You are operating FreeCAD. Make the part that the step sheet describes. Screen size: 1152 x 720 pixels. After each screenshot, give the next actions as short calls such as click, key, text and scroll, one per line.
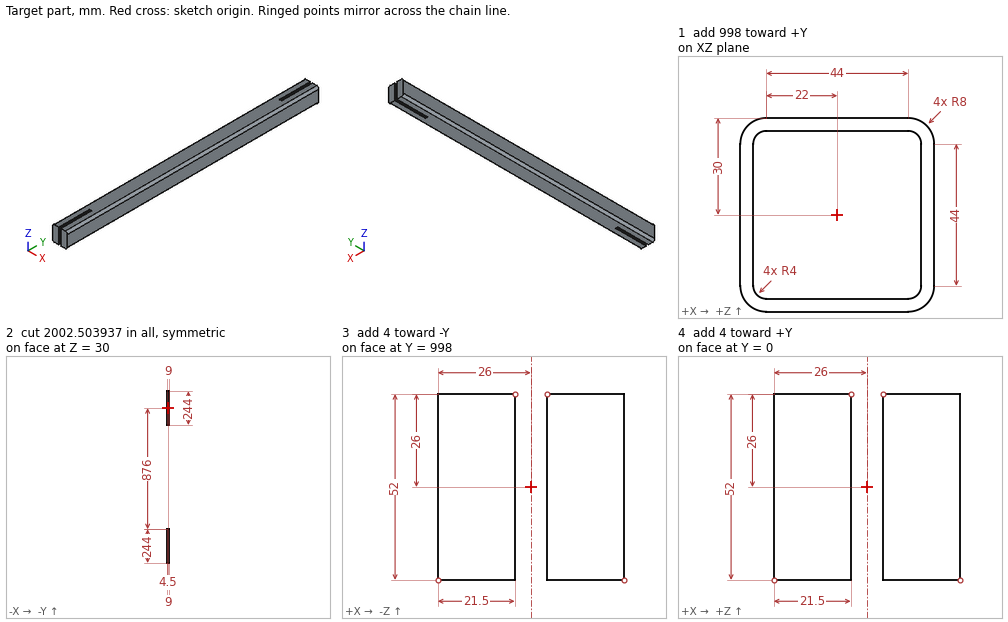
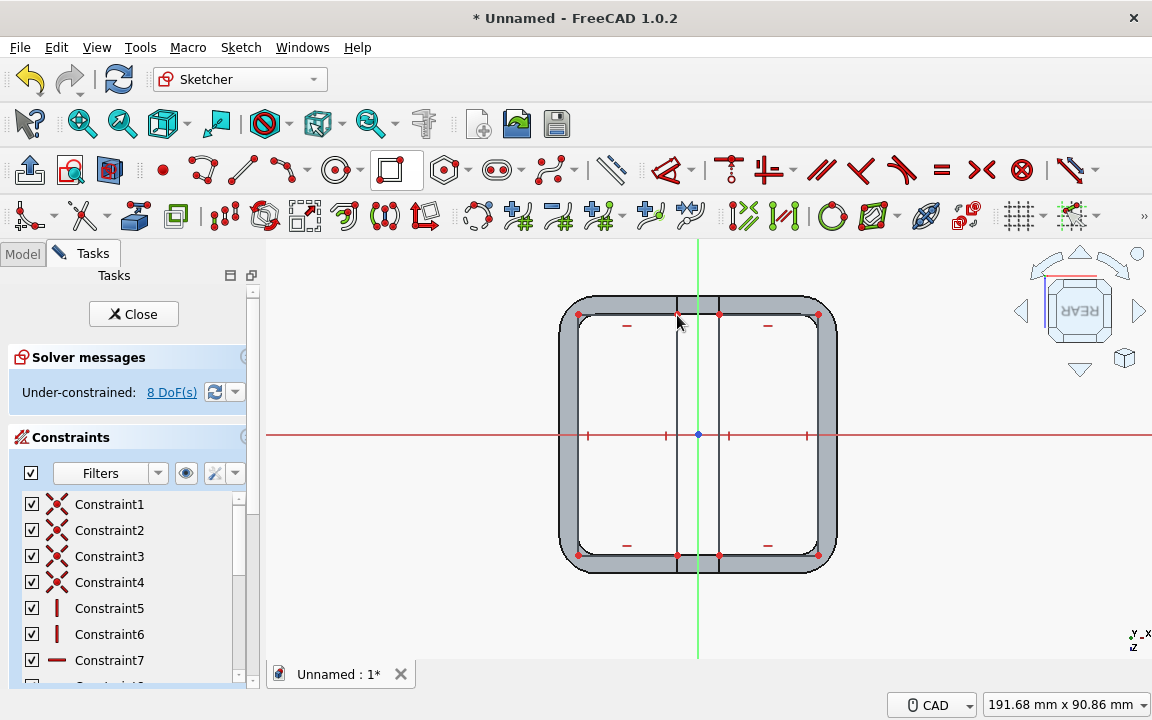
click(719, 315)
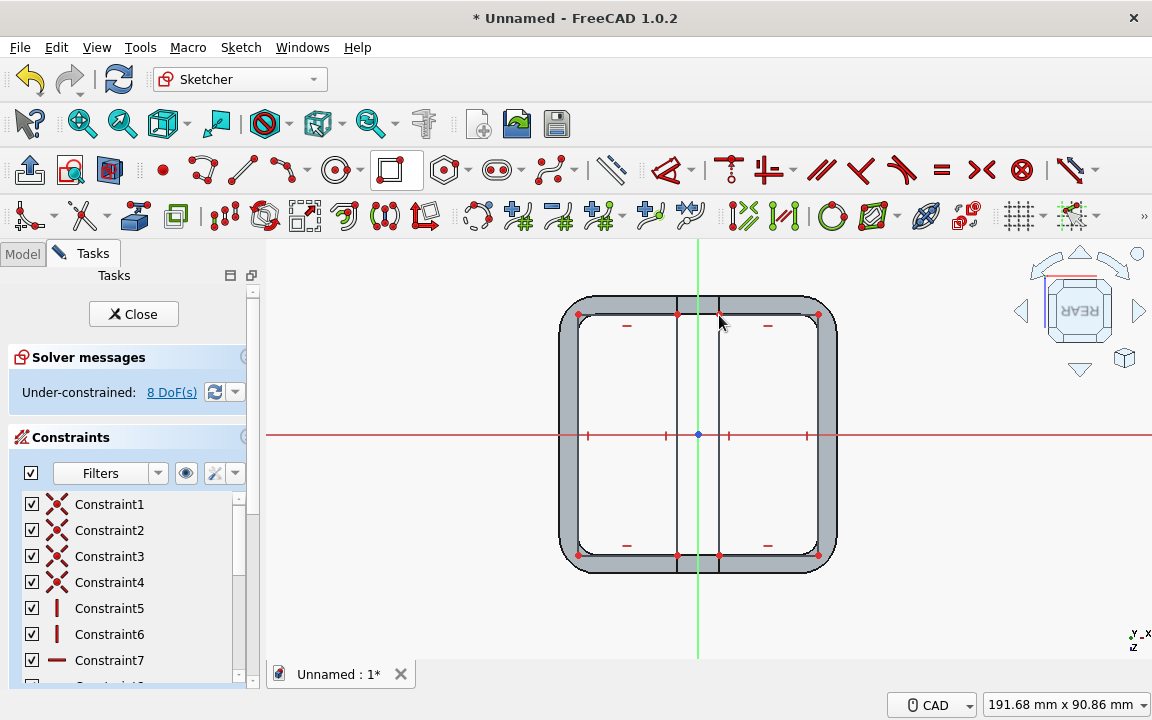
click(698, 605)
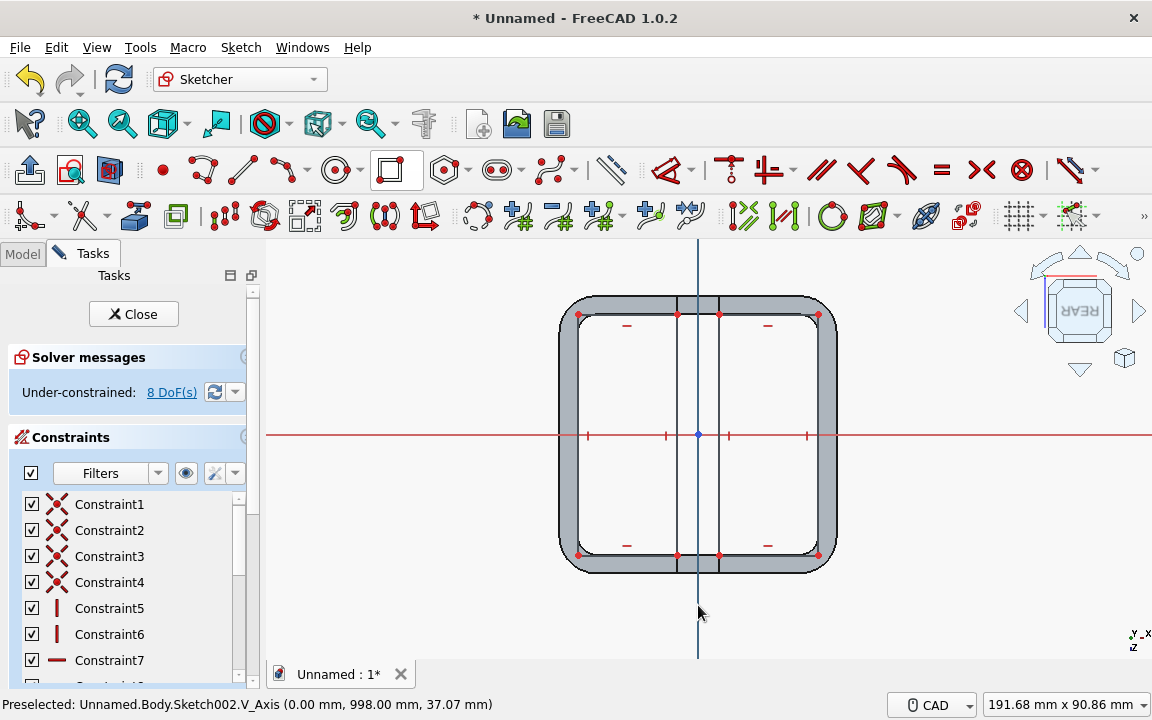
click(982, 170)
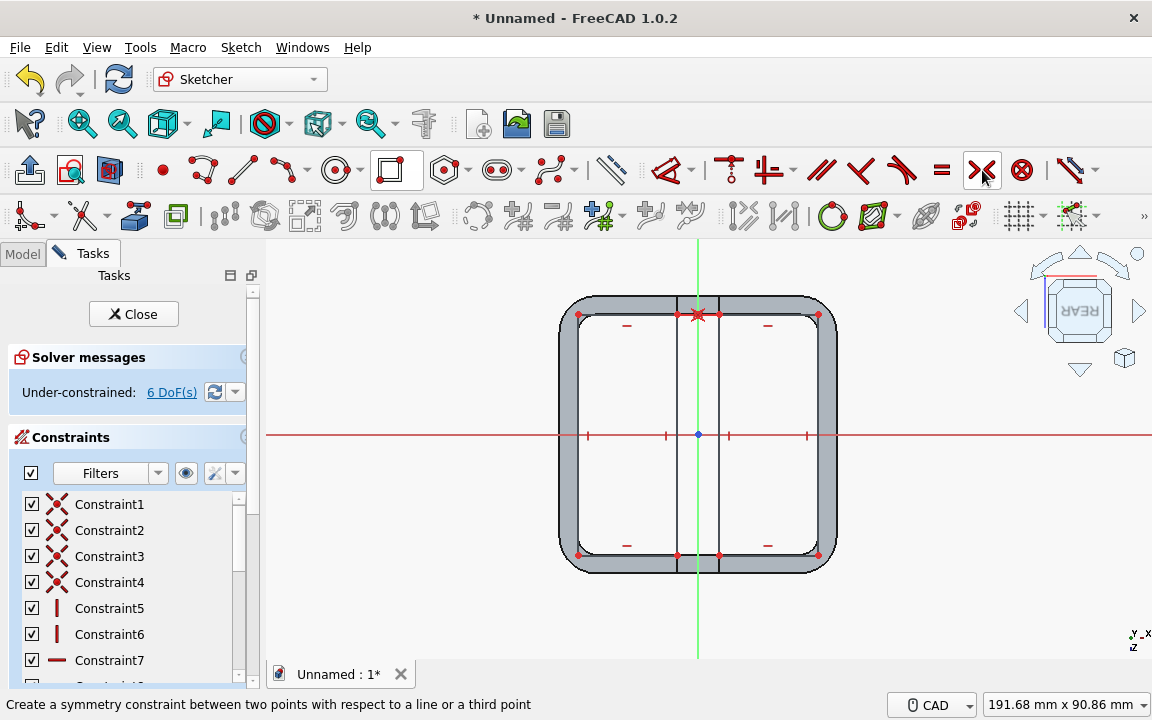
click(578, 556)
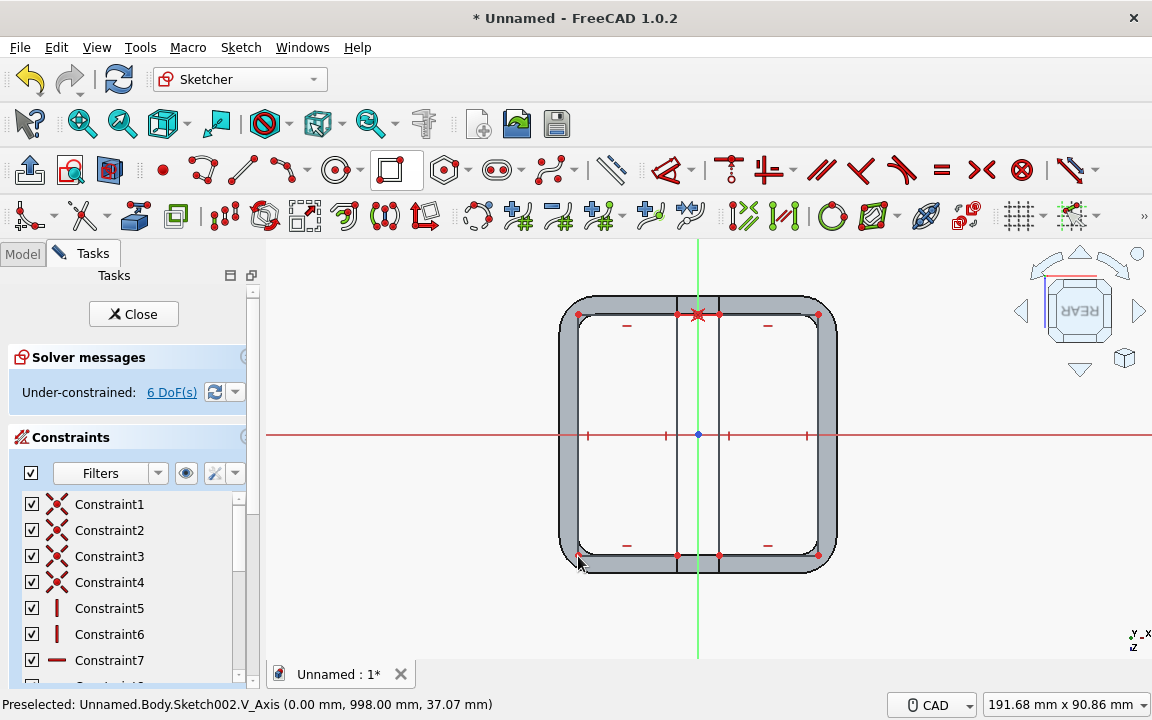
click(818, 556)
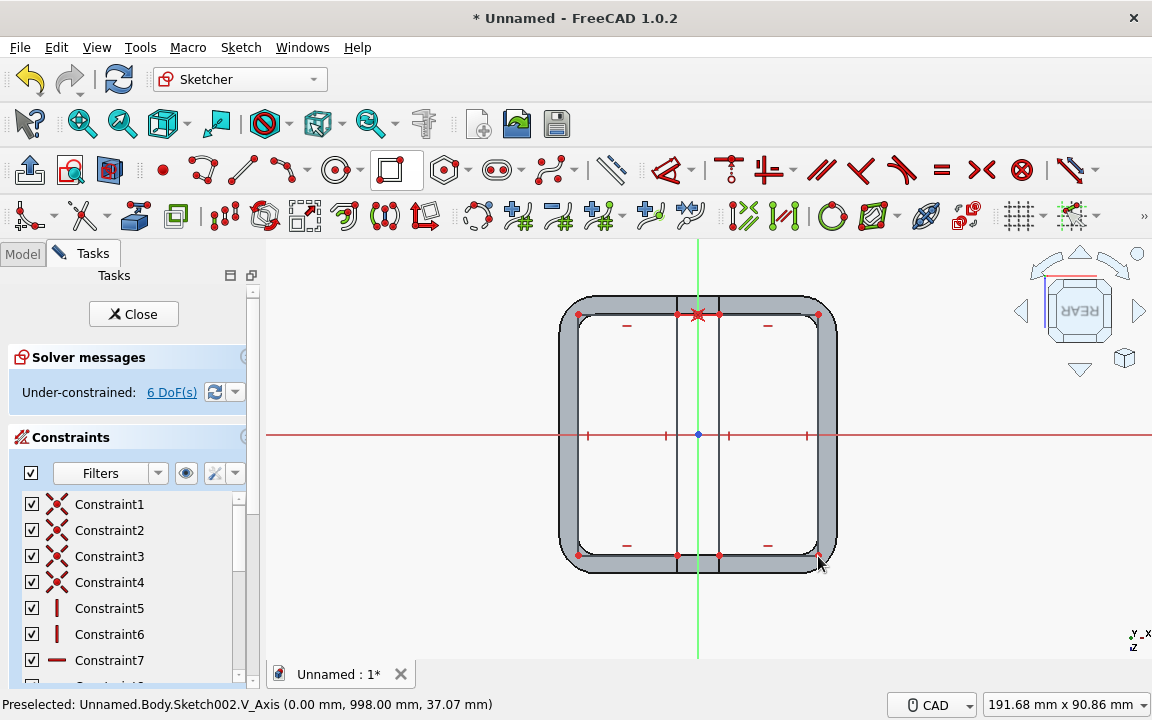
click(698, 605)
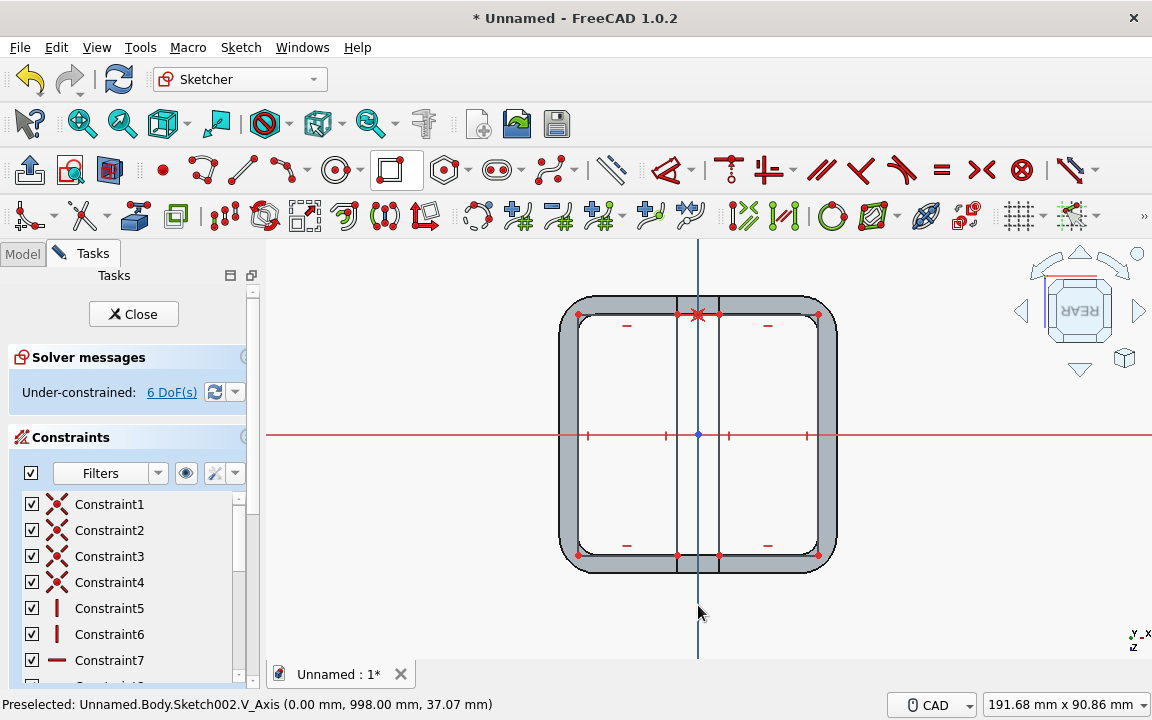
click(982, 170)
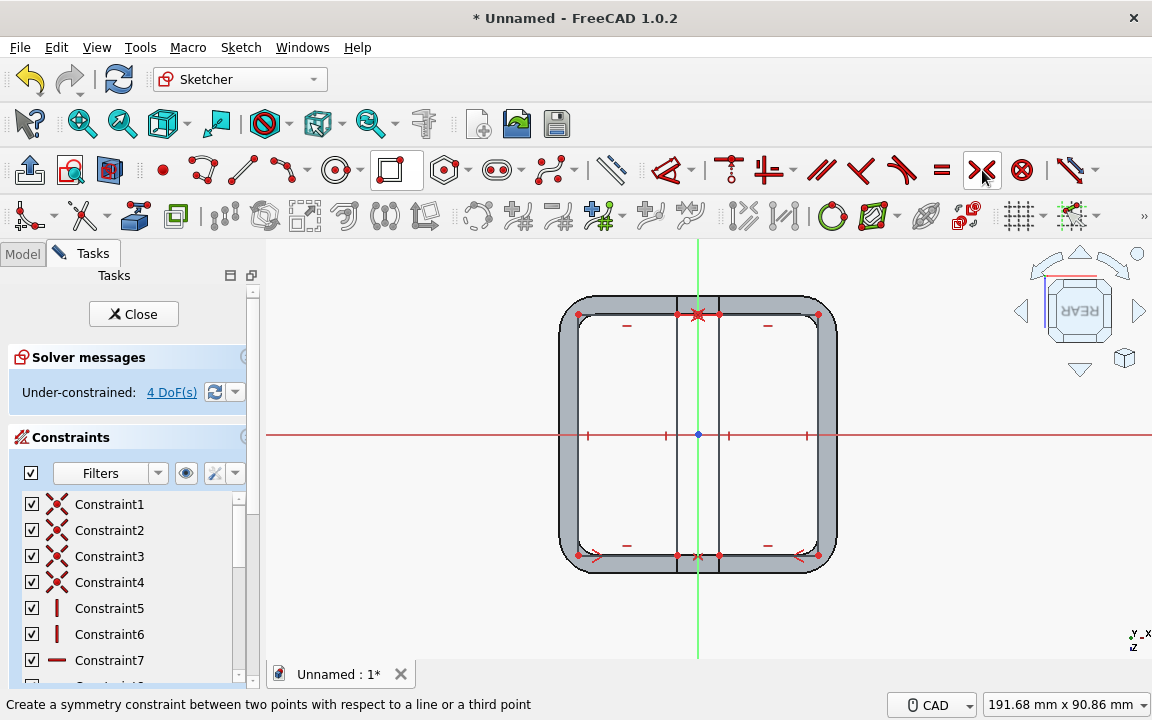
click(666, 170)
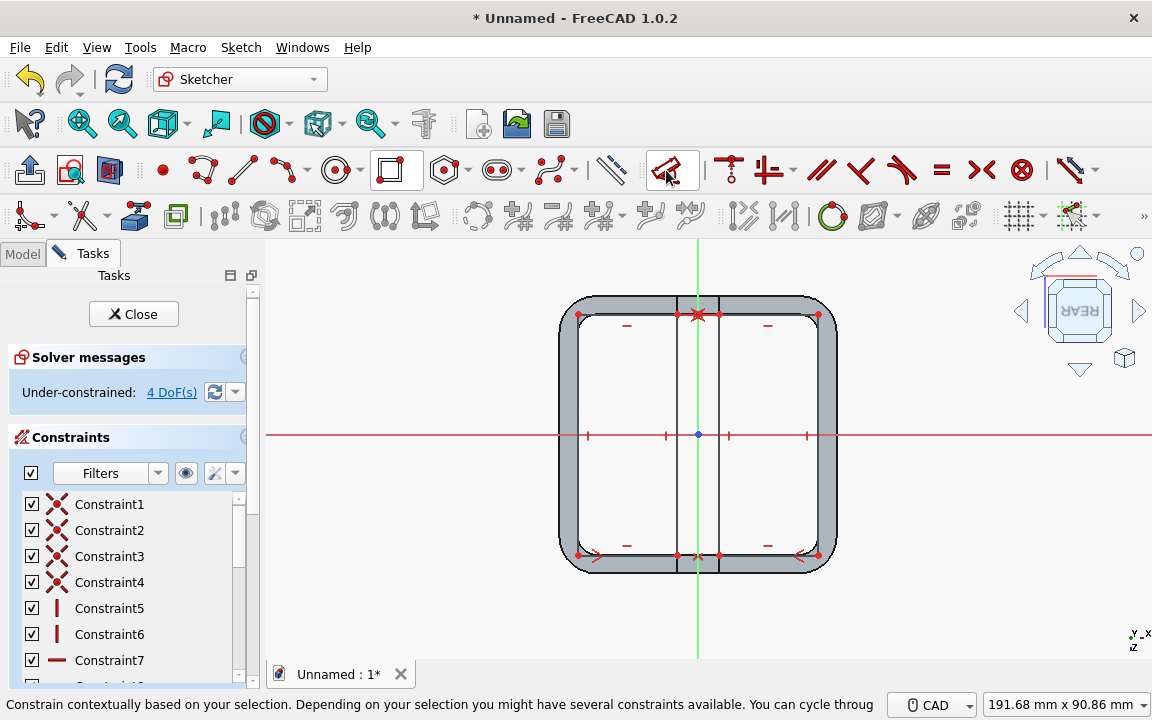
click(578, 387)
click(544, 380)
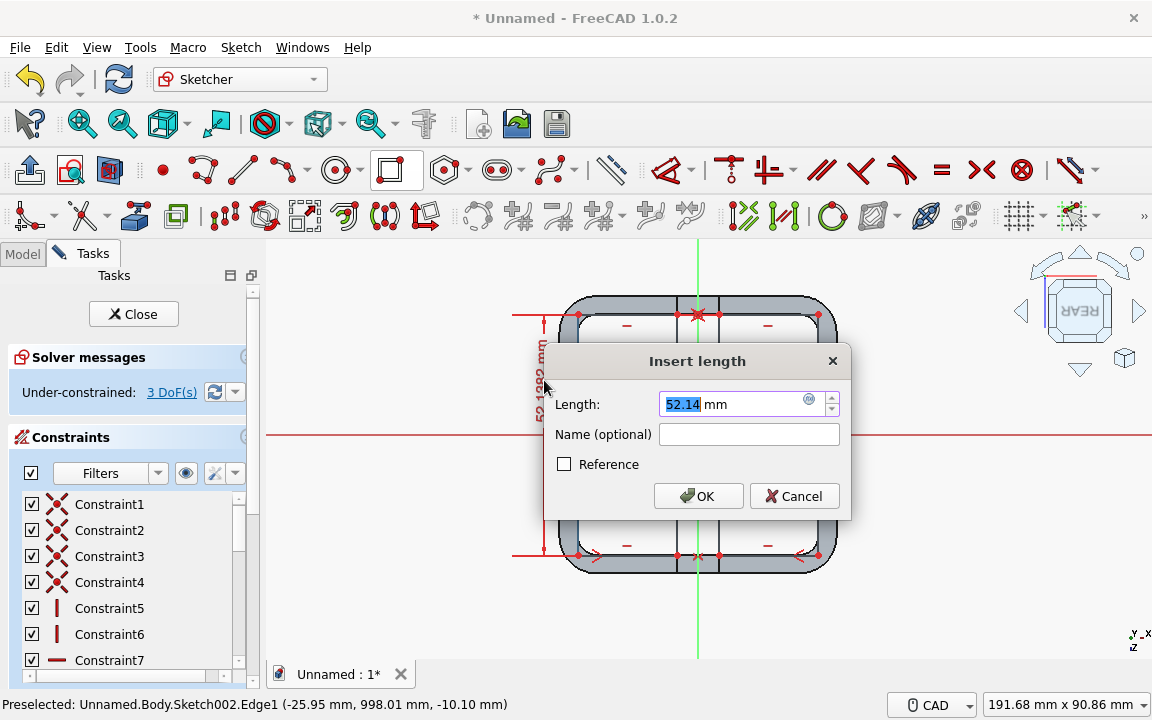
text(52)
key(Return)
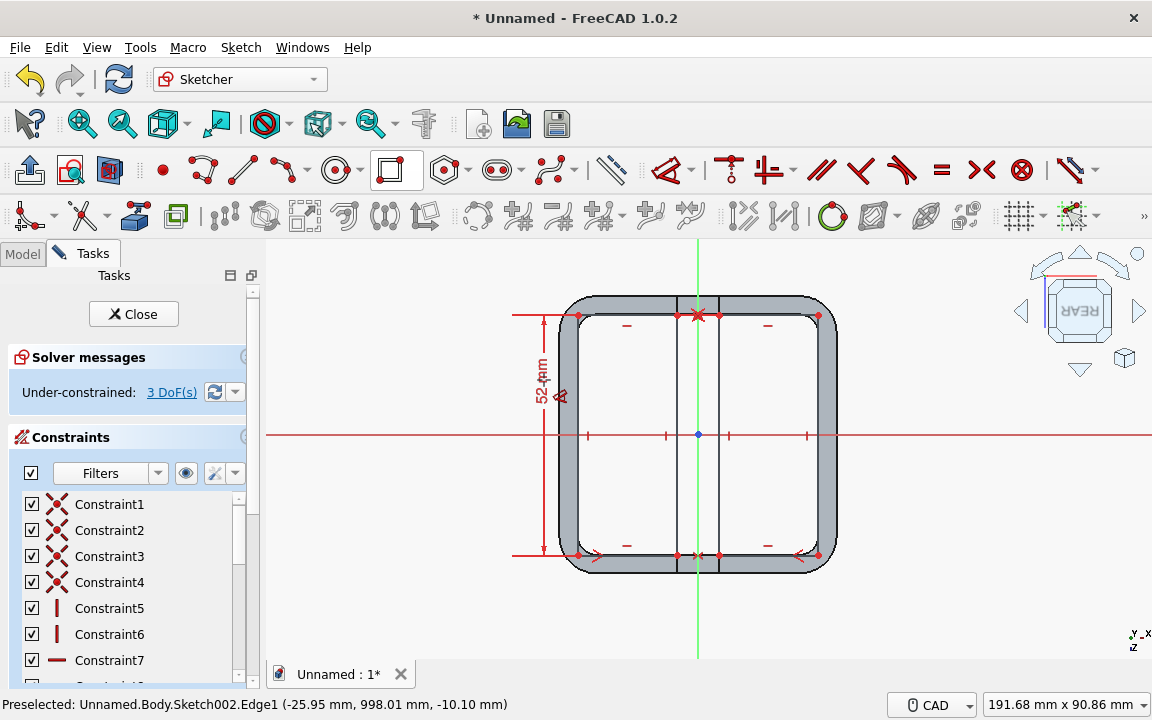
click(578, 315)
click(638, 281)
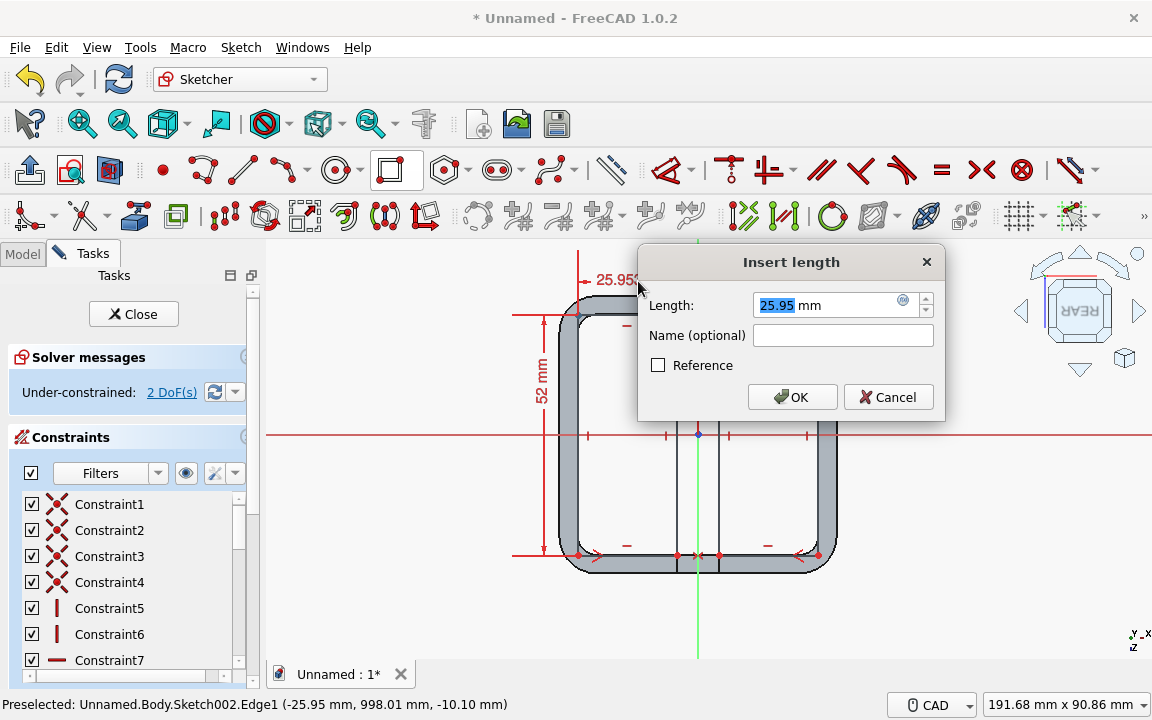
text(26)
key(Return)